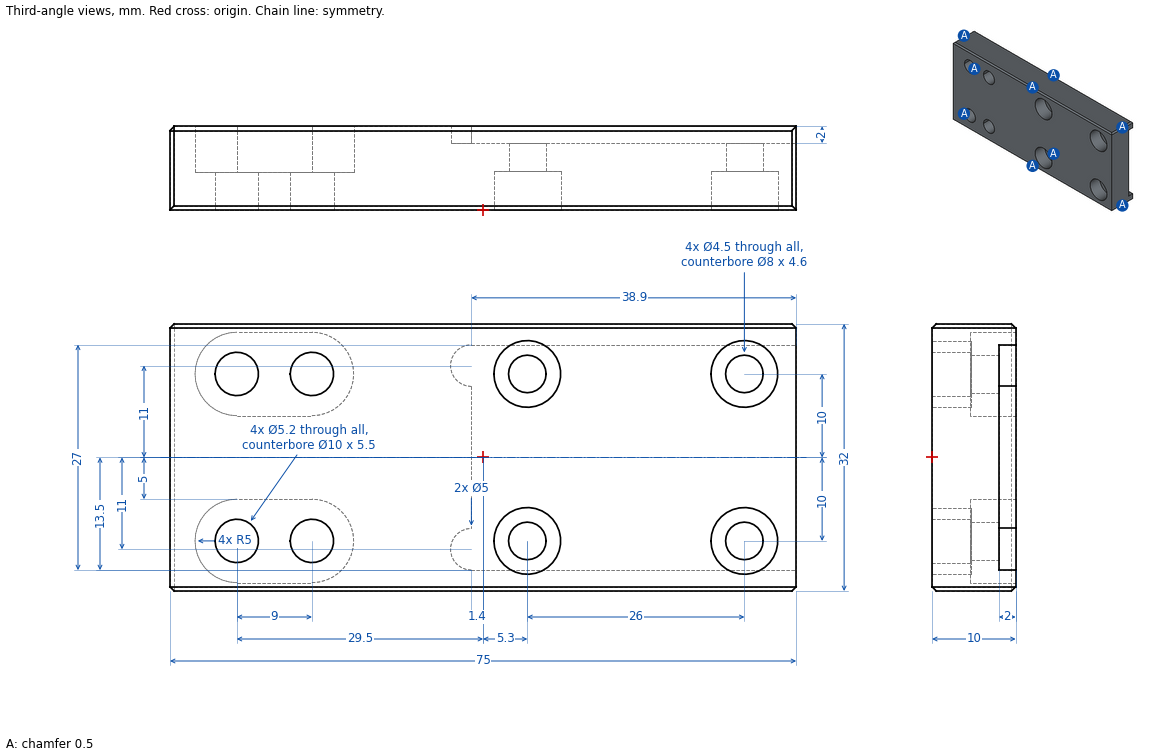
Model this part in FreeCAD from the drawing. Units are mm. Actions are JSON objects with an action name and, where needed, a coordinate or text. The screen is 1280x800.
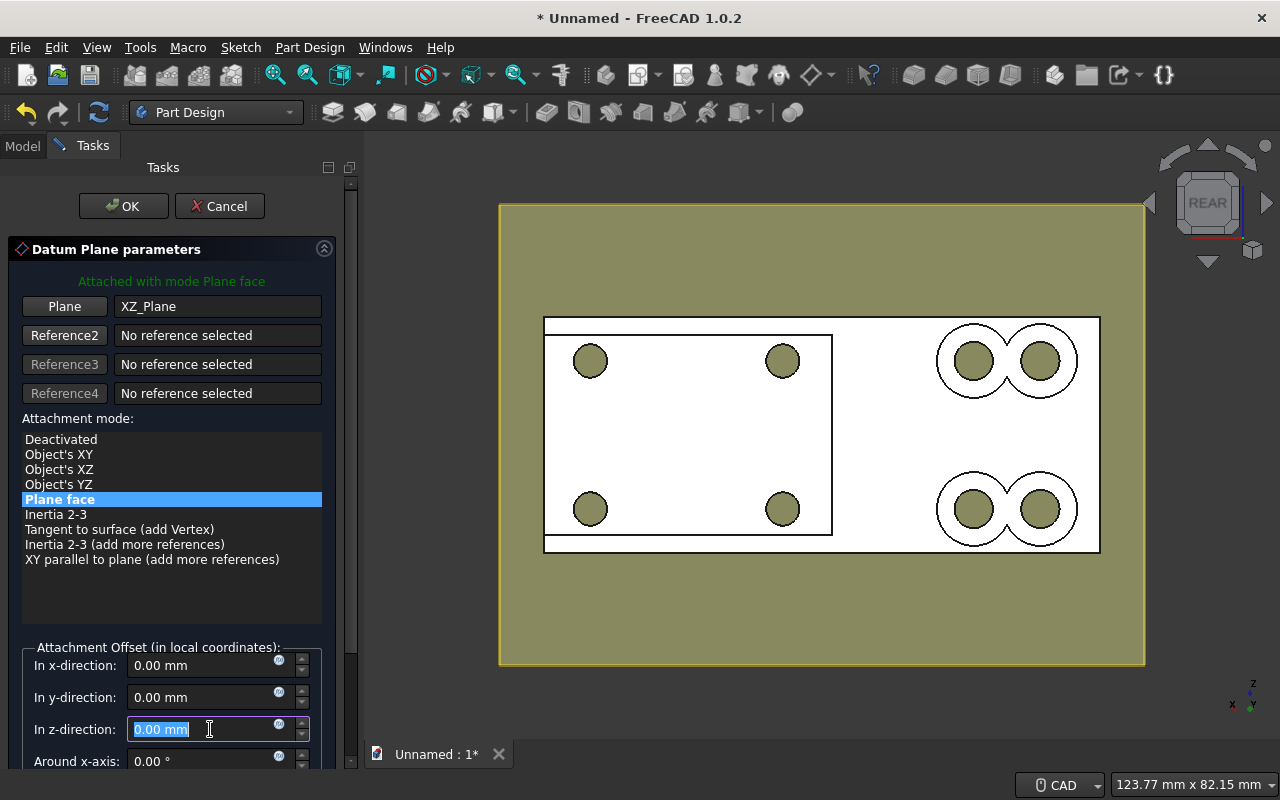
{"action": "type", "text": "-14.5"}
{"action": "key", "text": "Tab"}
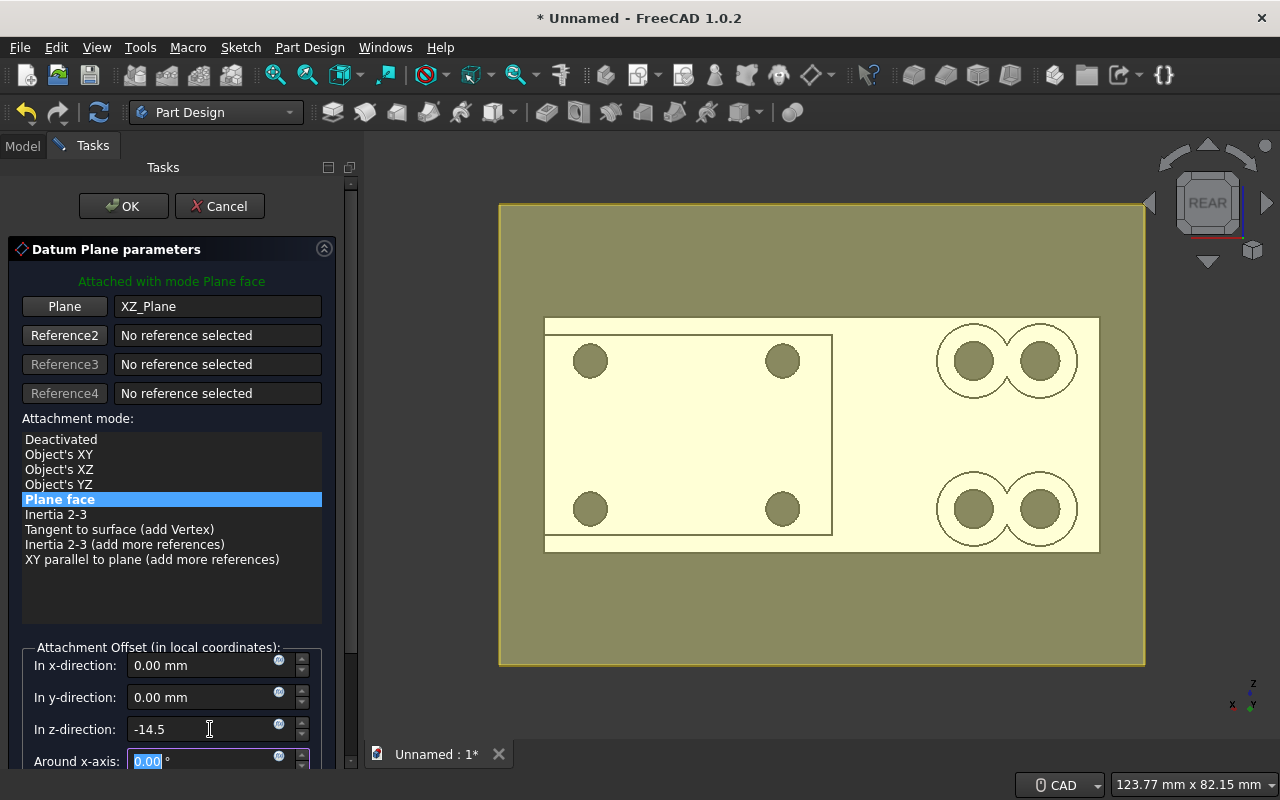
{"action": "left_click", "coordinate": [124, 206]}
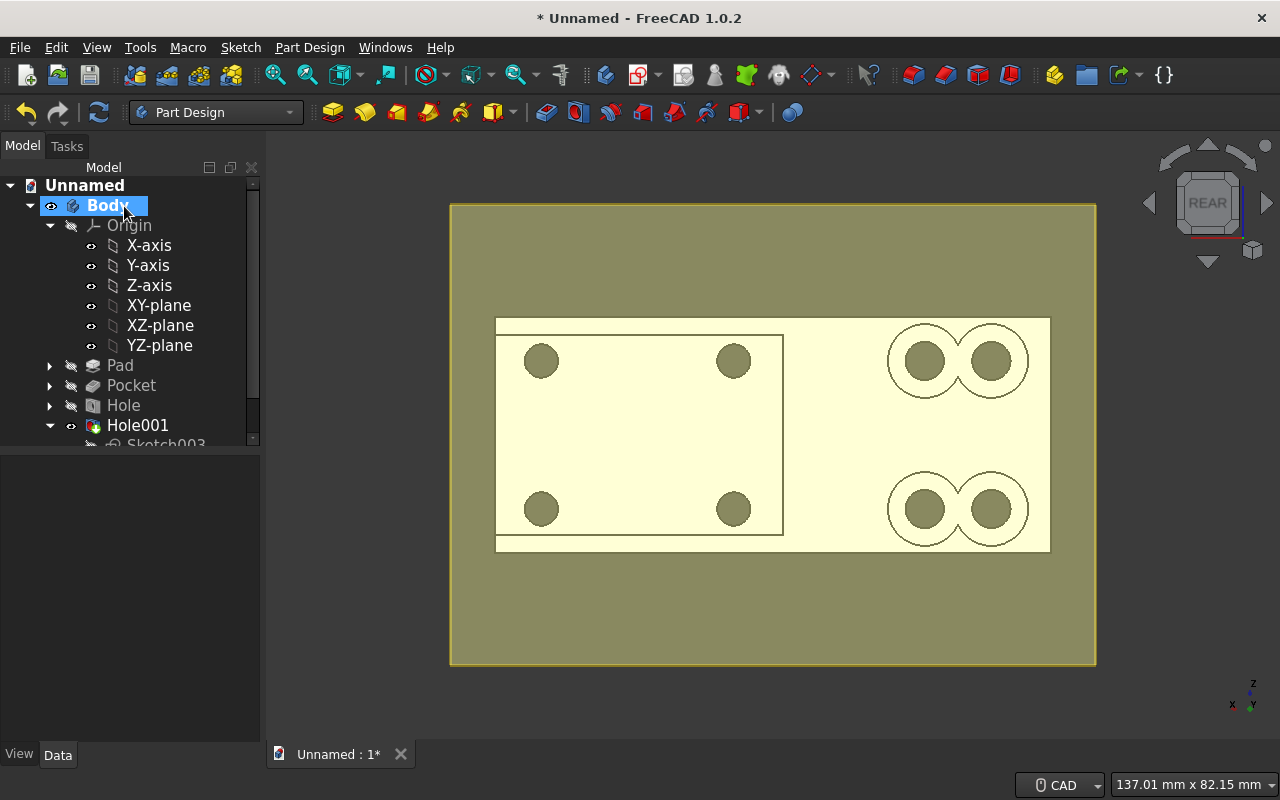
{"action": "scroll", "coordinate": [100, 321], "scroll_direction": "down", "scroll_amount": 3}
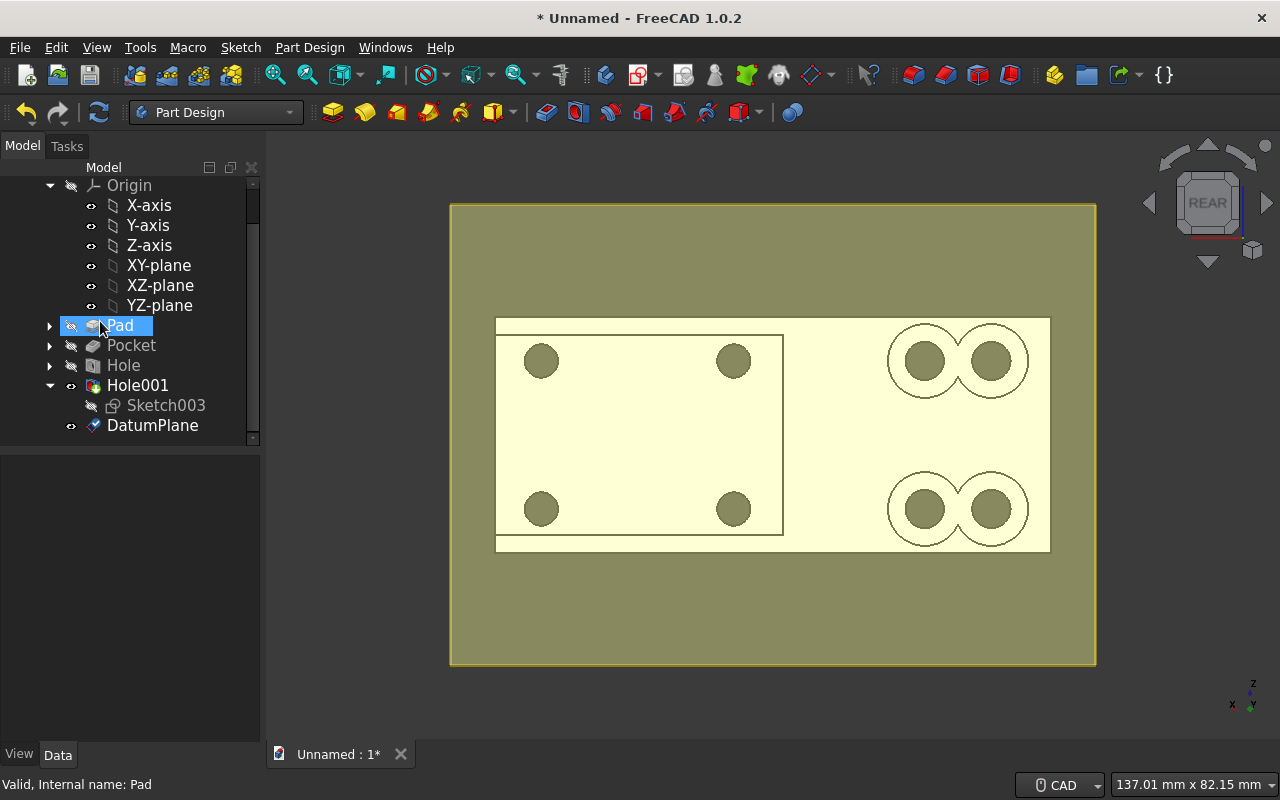
{"action": "left_click", "coordinate": [116, 426]}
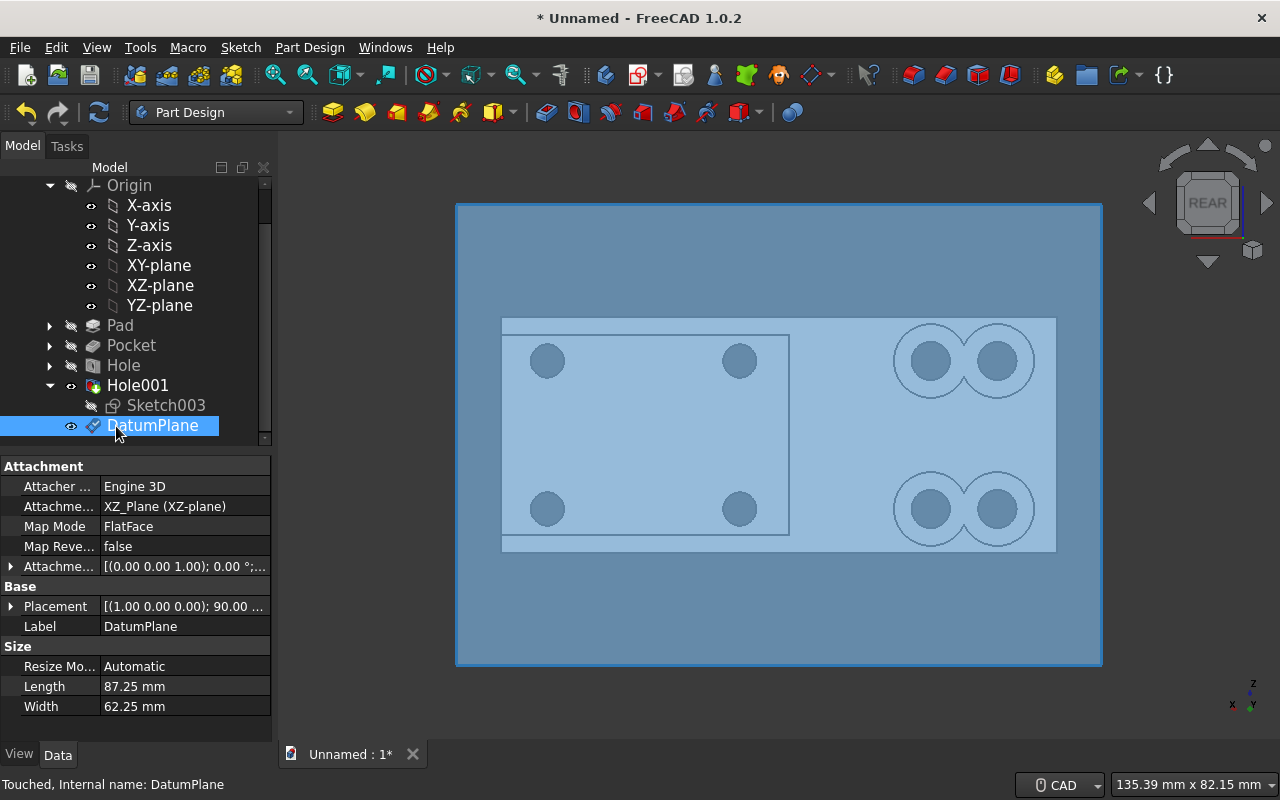
{"action": "left_click", "coordinate": [638, 76]}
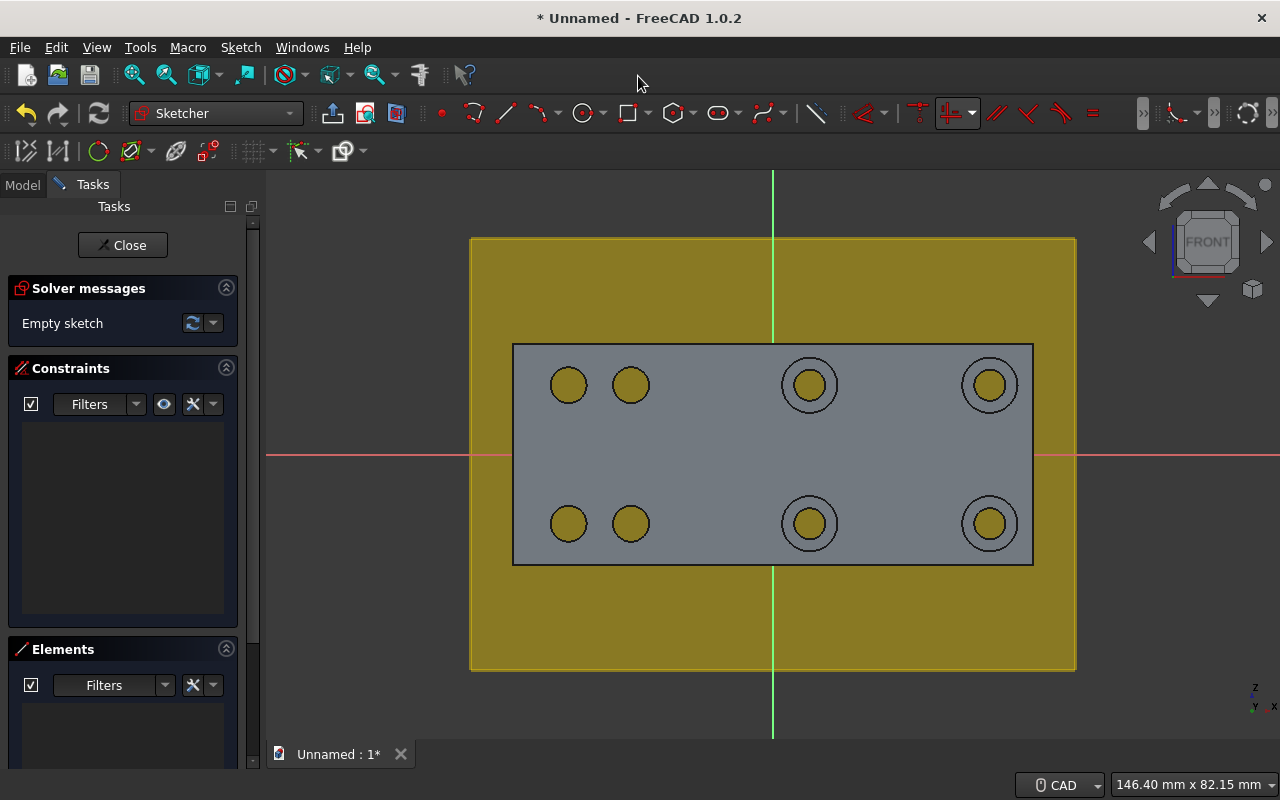
{"action": "left_click", "coordinate": [398, 114]}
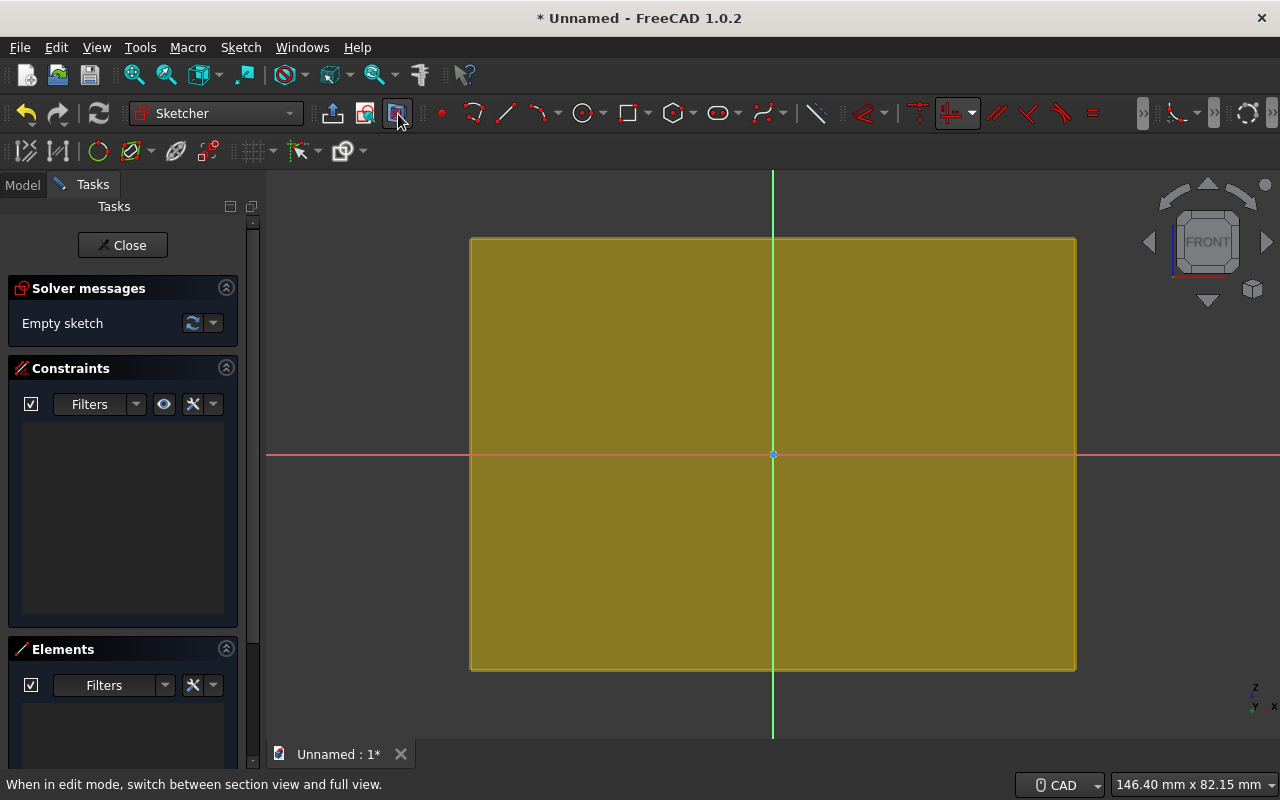
{"action": "scroll", "coordinate": [592, 455], "scroll_direction": "up", "scroll_amount": 3}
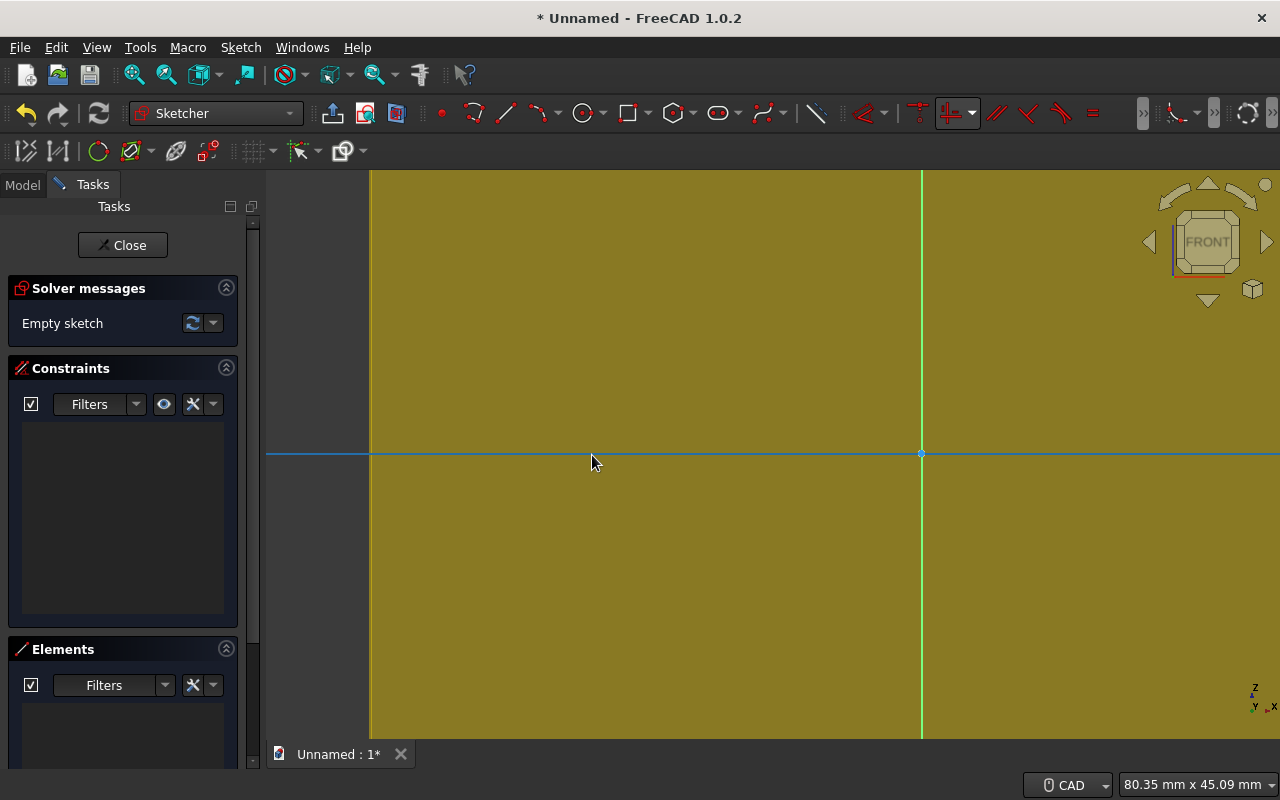
{"action": "left_click", "coordinate": [718, 114]}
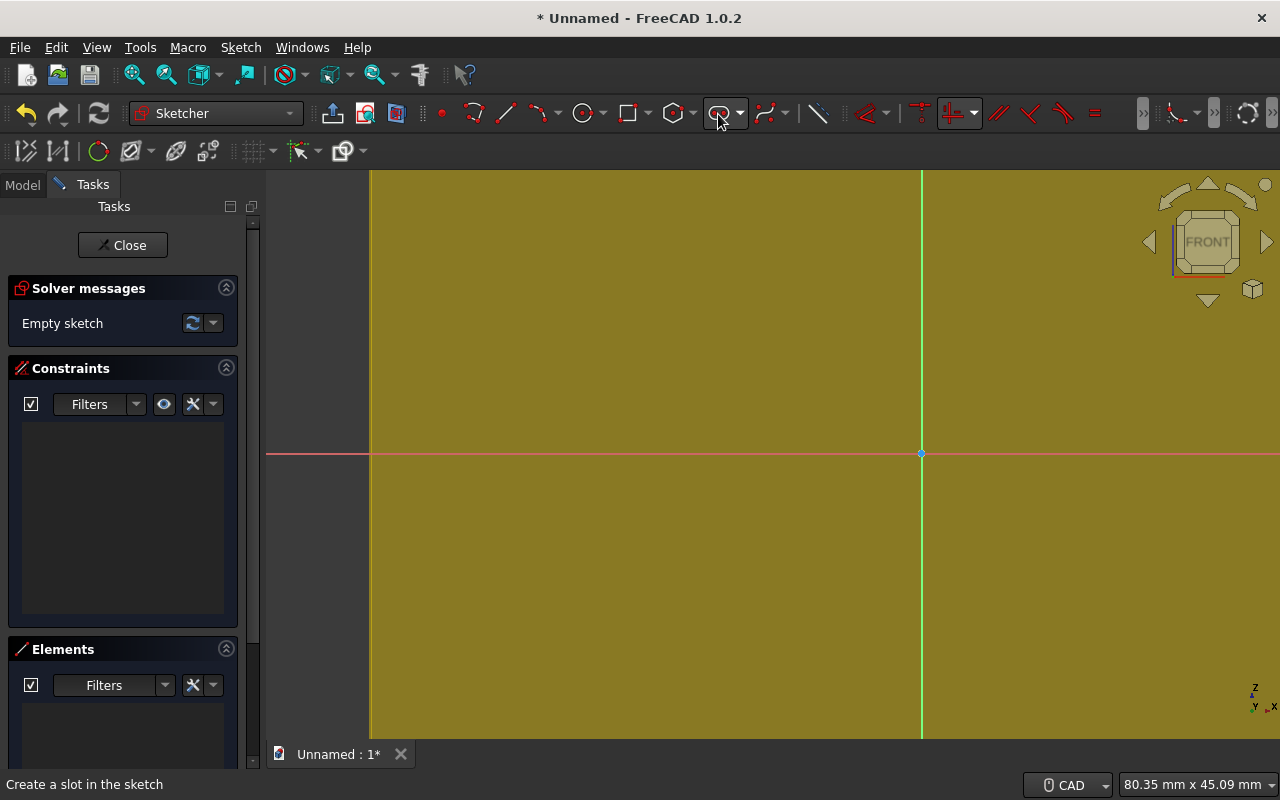
{"action": "left_click", "coordinate": [549, 580]}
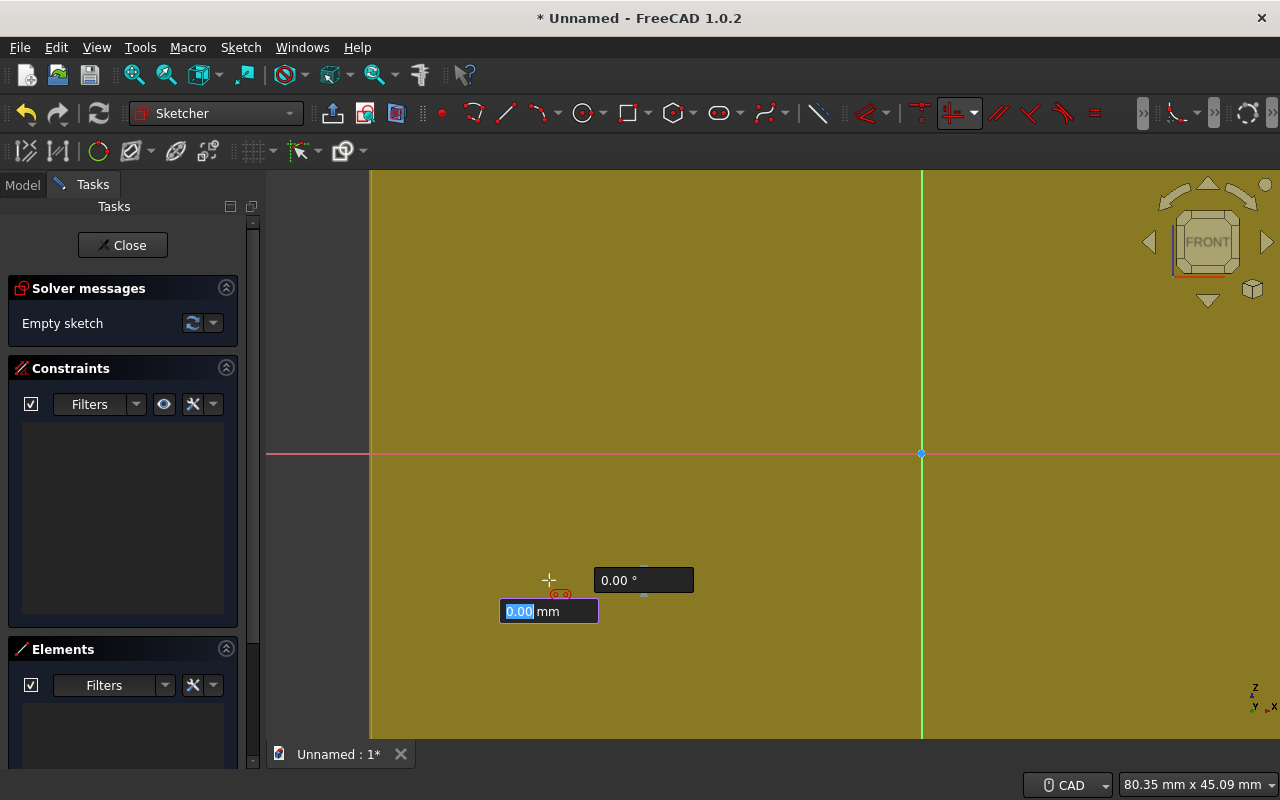
{"action": "left_click", "coordinate": [663, 580]}